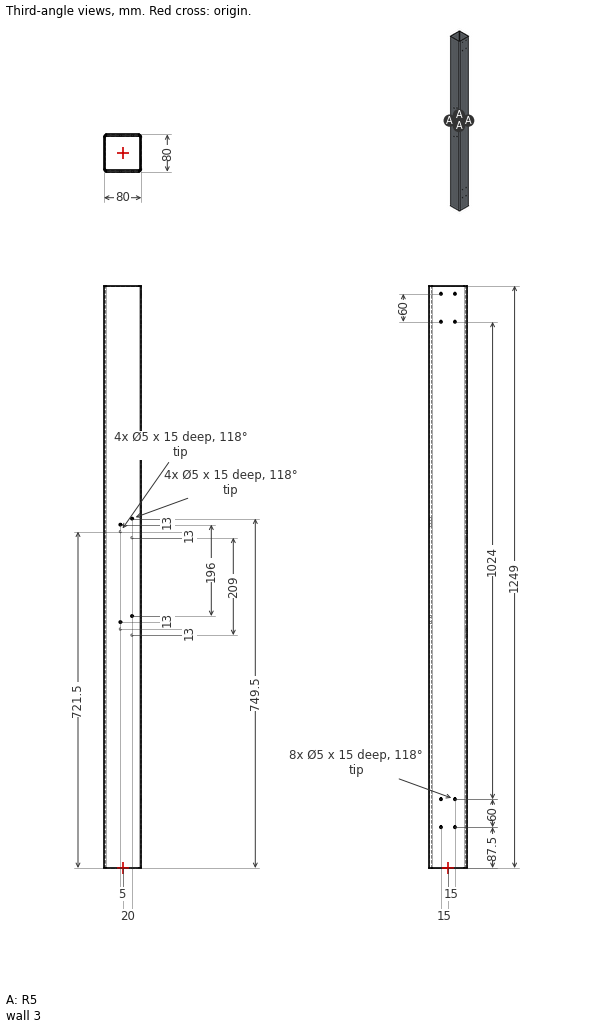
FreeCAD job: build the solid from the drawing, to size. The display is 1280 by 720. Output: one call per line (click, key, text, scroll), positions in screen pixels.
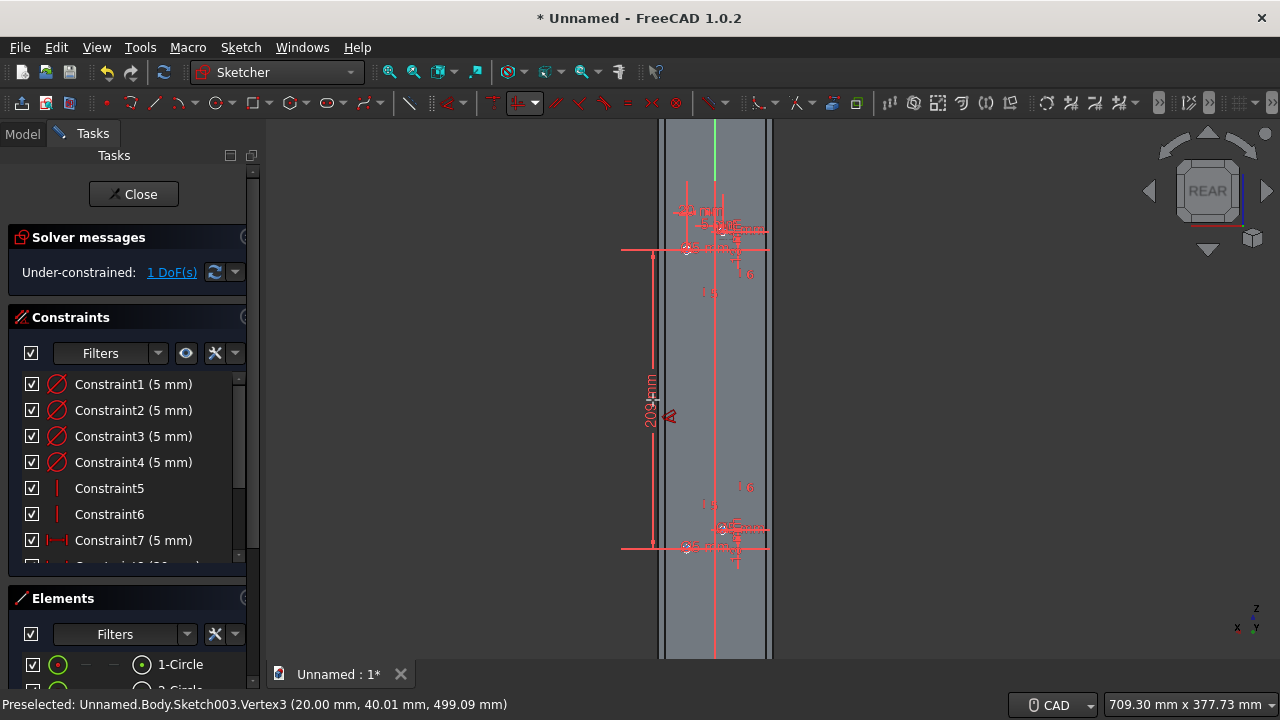
click(723, 232)
click(757, 431)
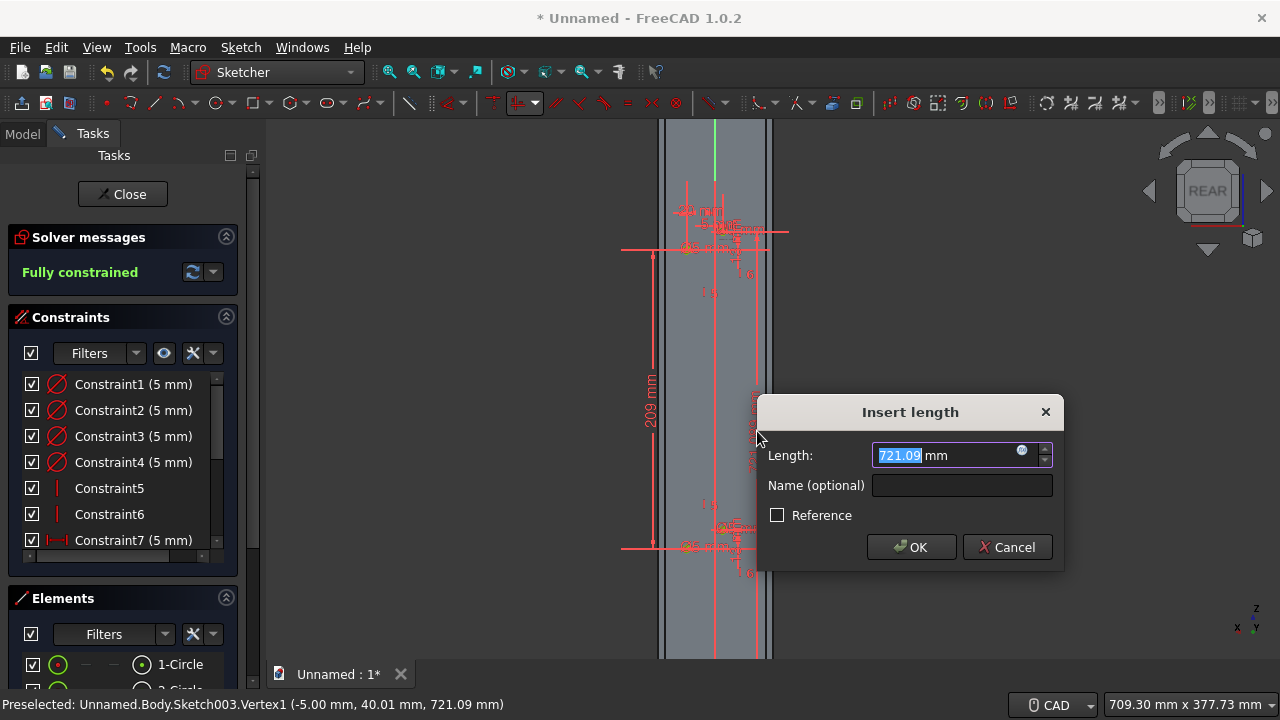
text(721.5)
key(Return)
key(Escape)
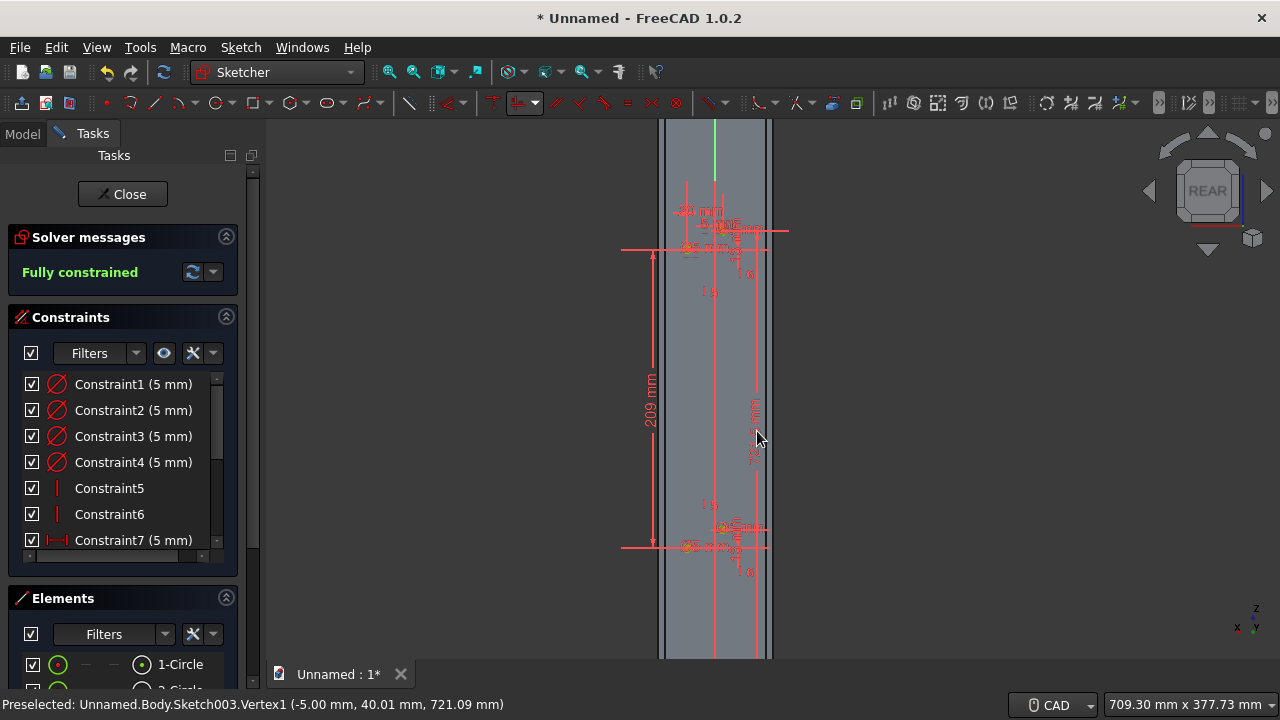
click(123, 194)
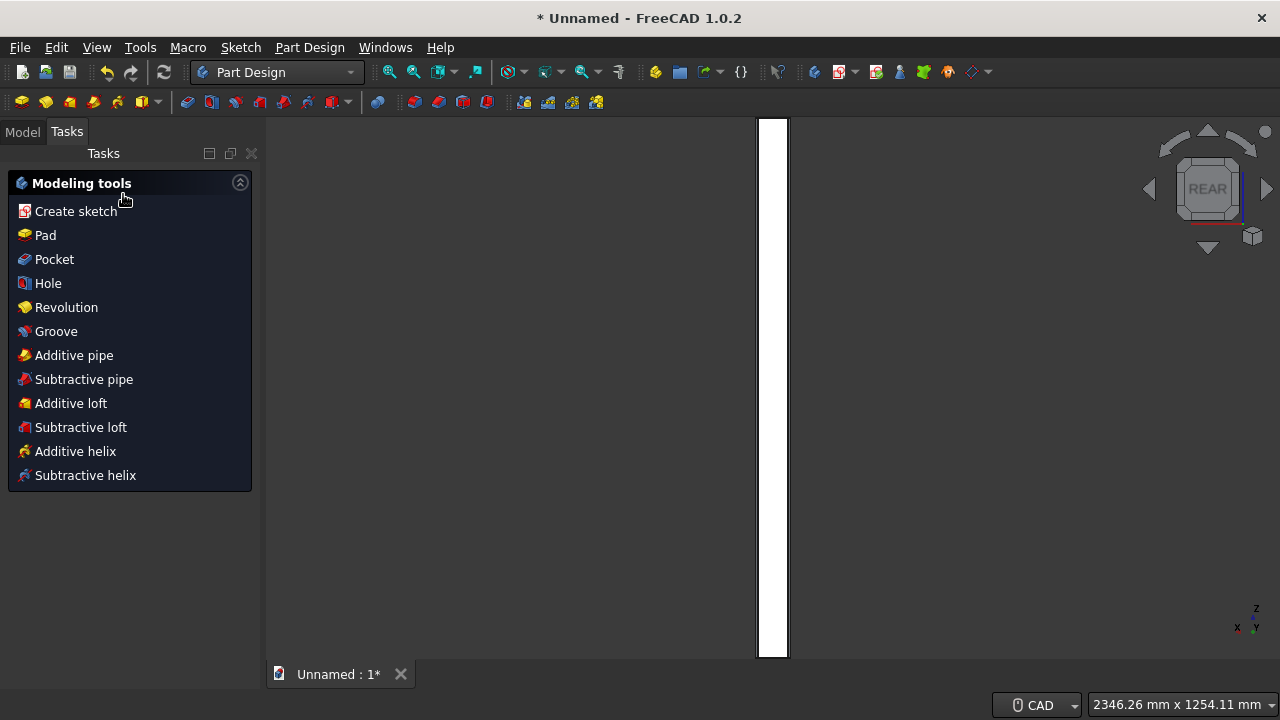
click(212, 102)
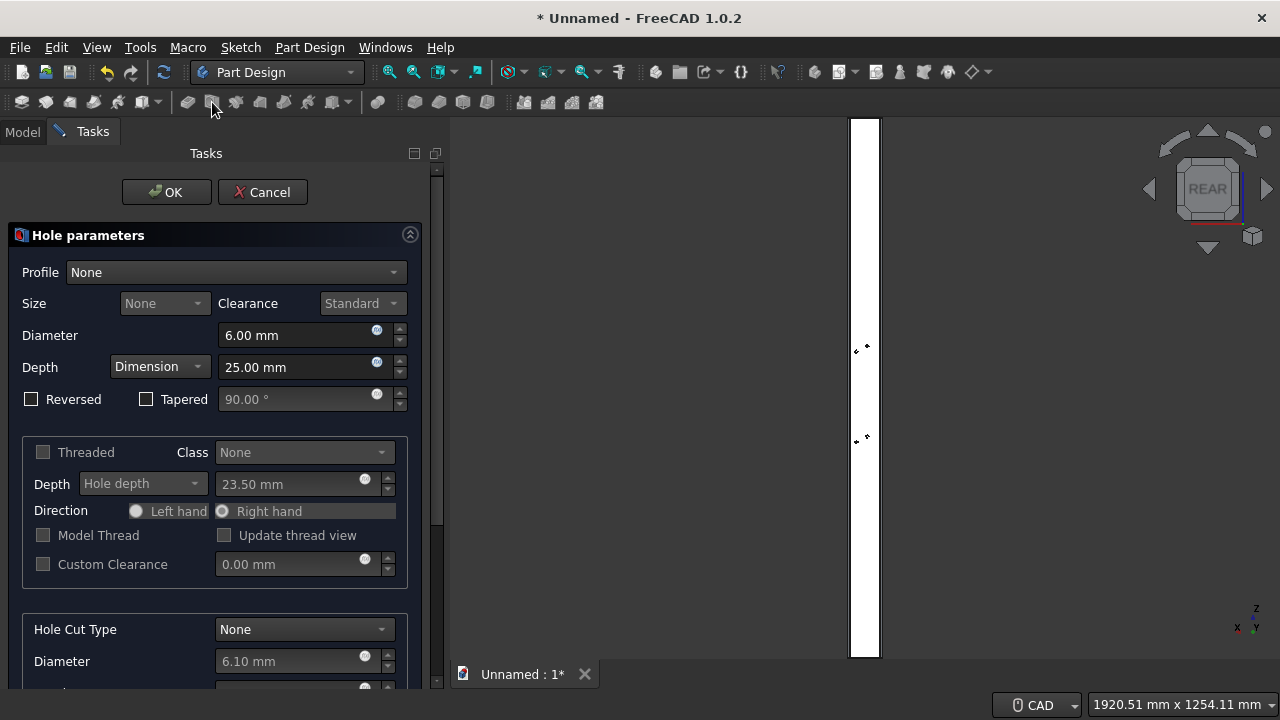
triple_click(305, 335)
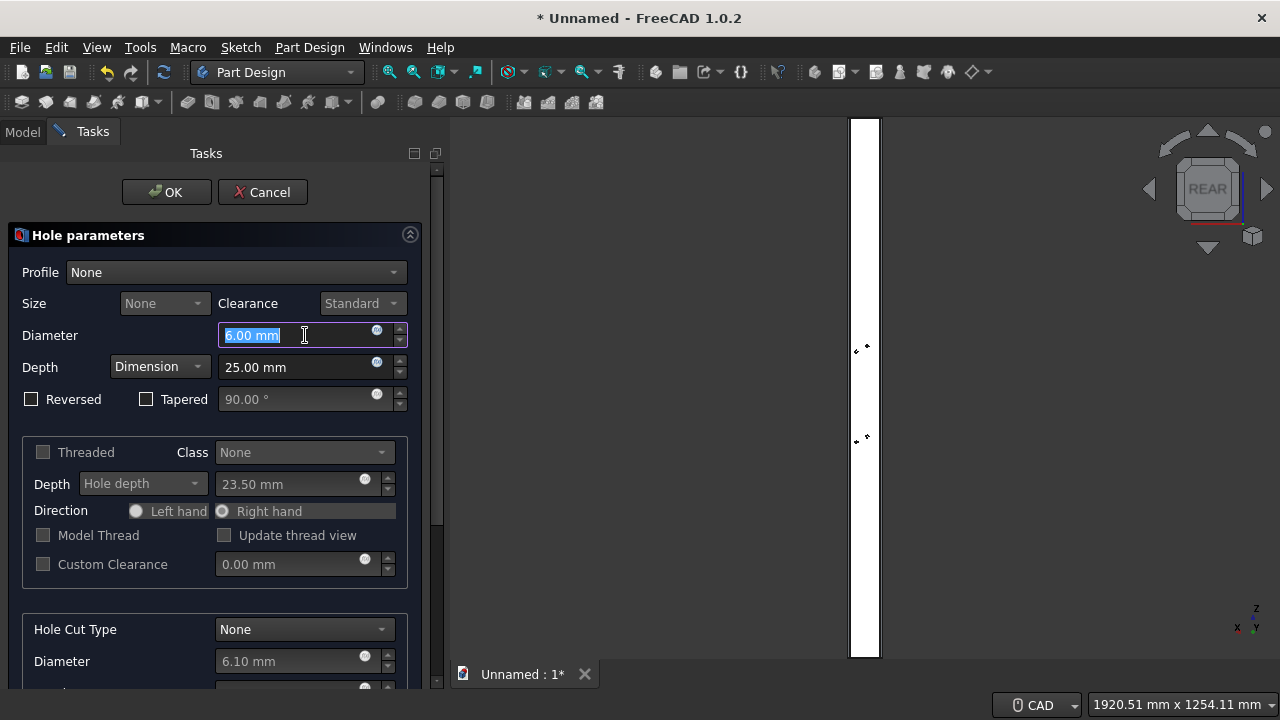
text(5)
key(Tab)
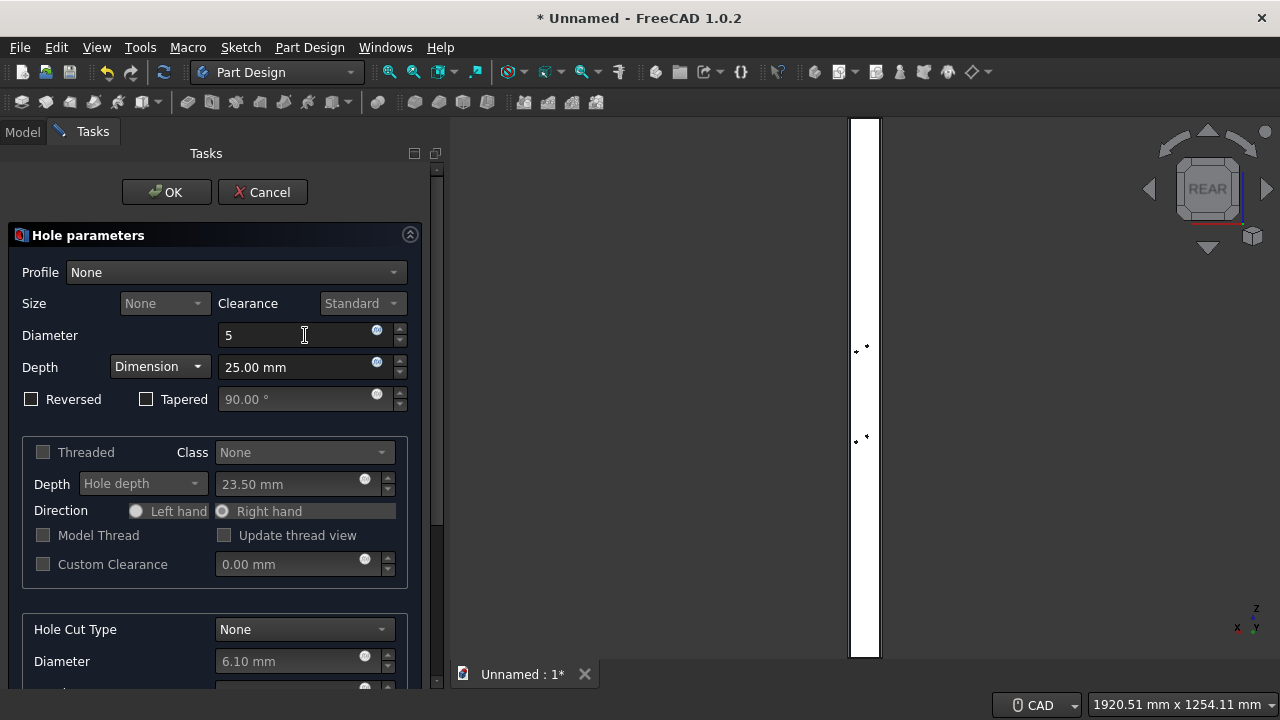
triple_click(305, 367)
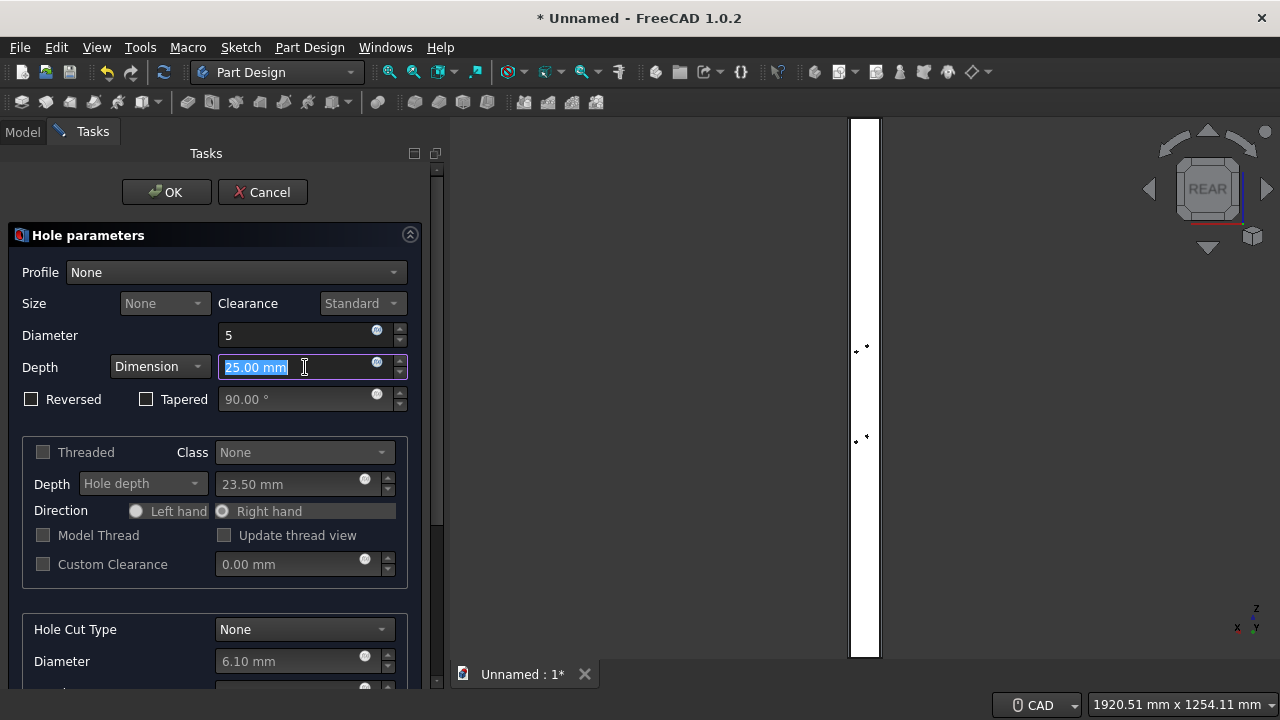
text(15)
key(Tab)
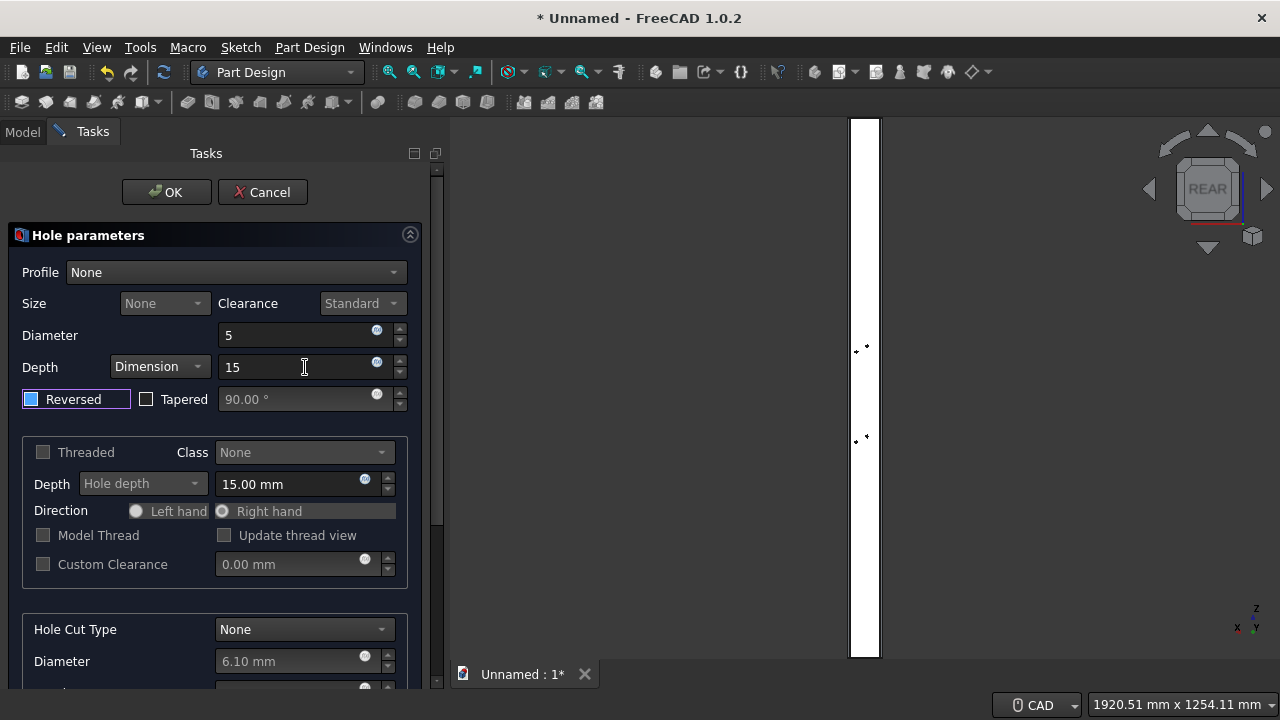
click(167, 192)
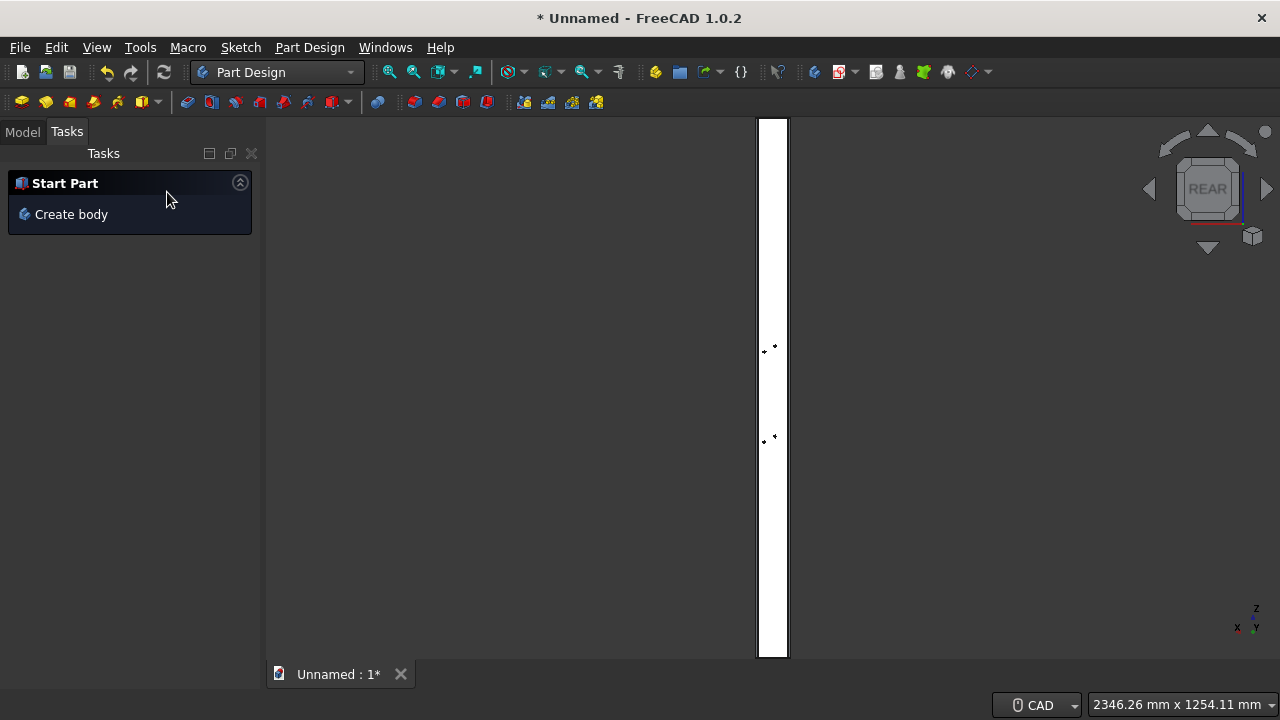
key(0)